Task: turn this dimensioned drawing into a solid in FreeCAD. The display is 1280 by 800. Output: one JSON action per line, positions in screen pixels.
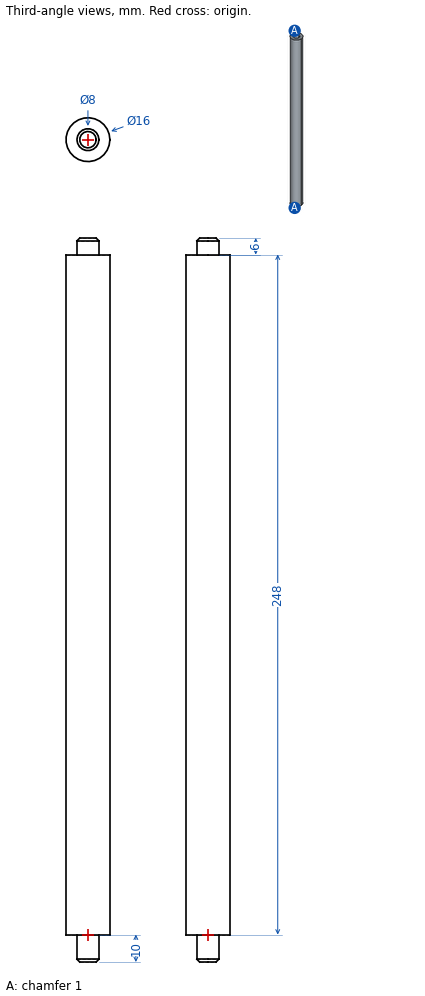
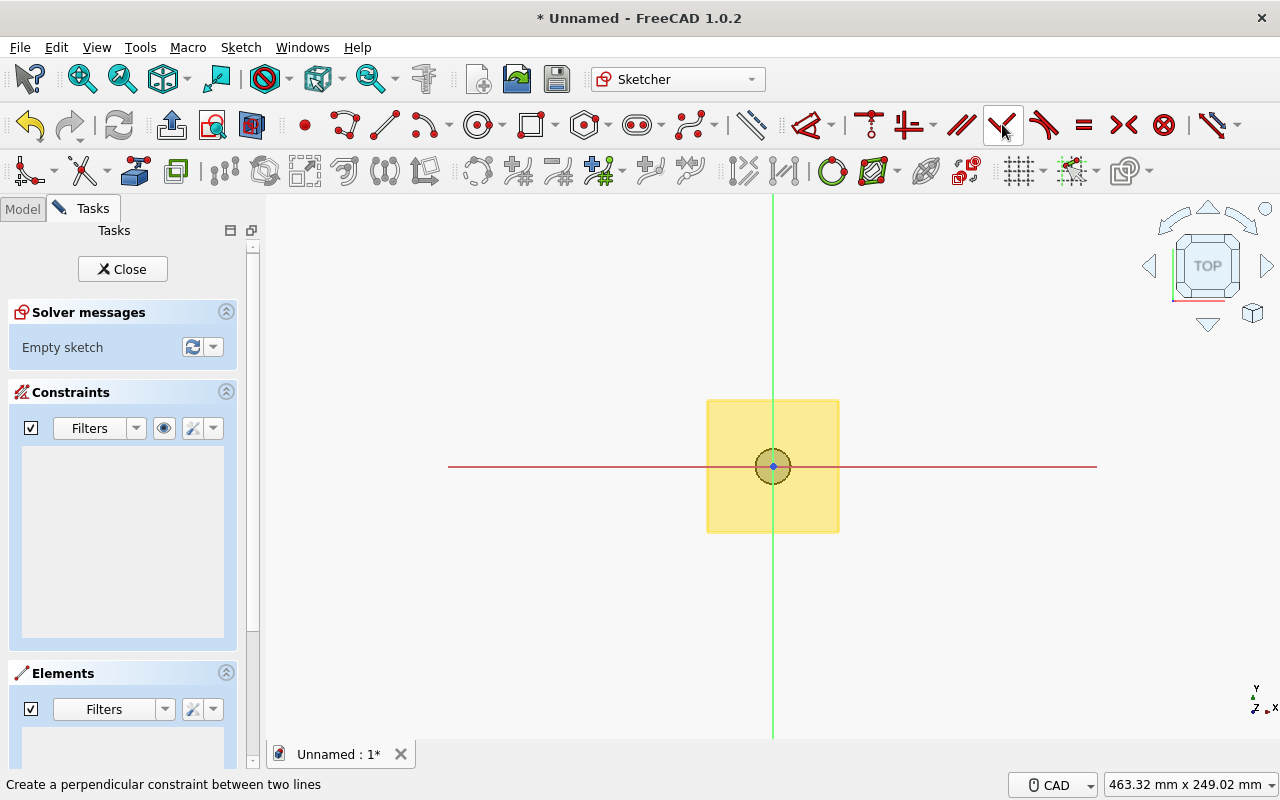
{"action": "scroll", "coordinate": [777, 466], "scroll_direction": "up", "scroll_amount": 15}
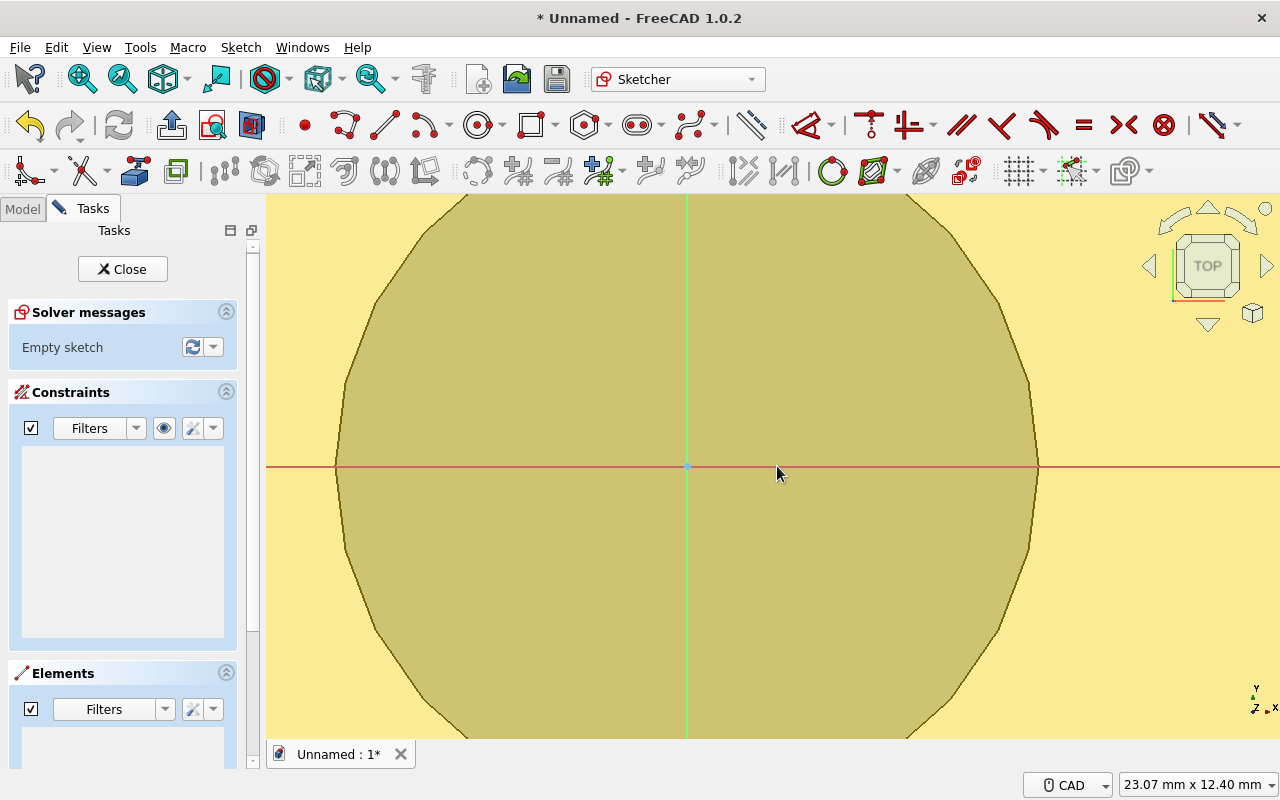
{"action": "key", "text": "g c"}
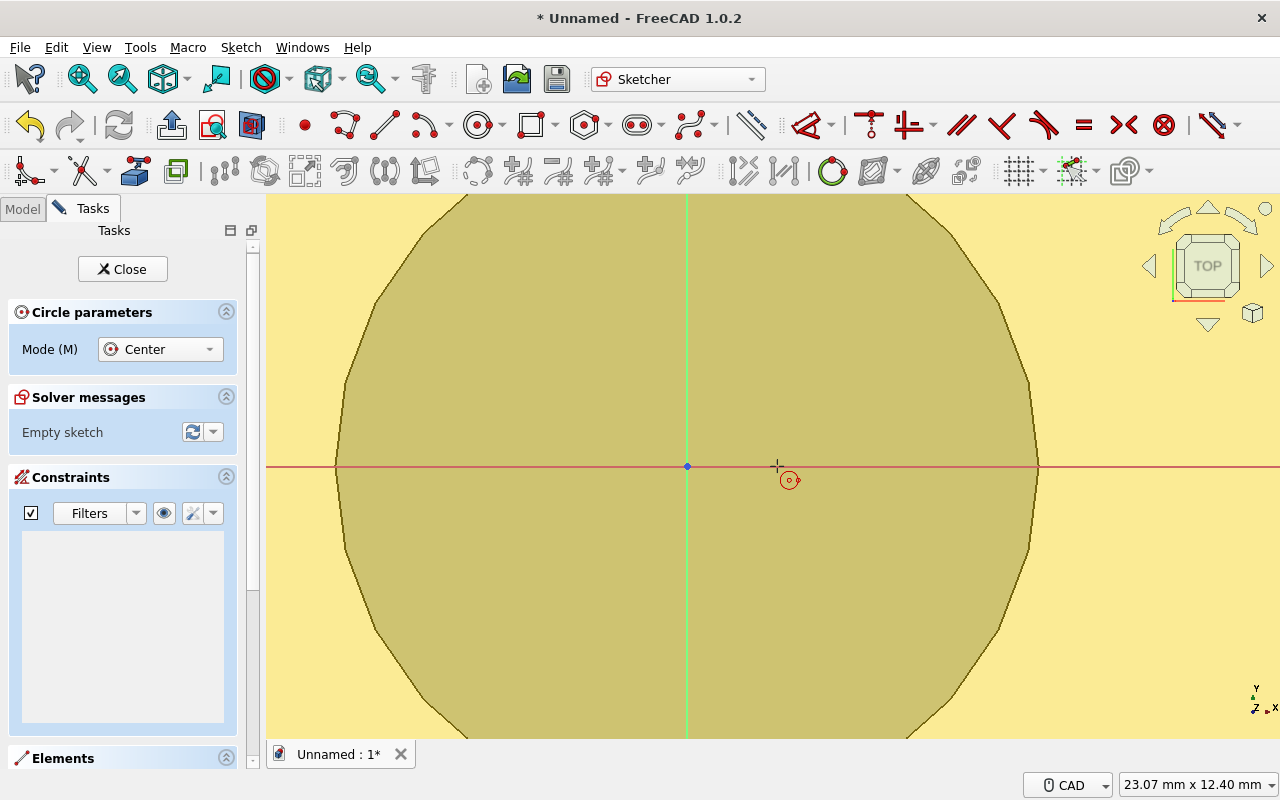
{"action": "left_click", "coordinate": [687, 466]}
{"action": "left_click", "coordinate": [811, 342]}
{"action": "key", "text": "Escape"}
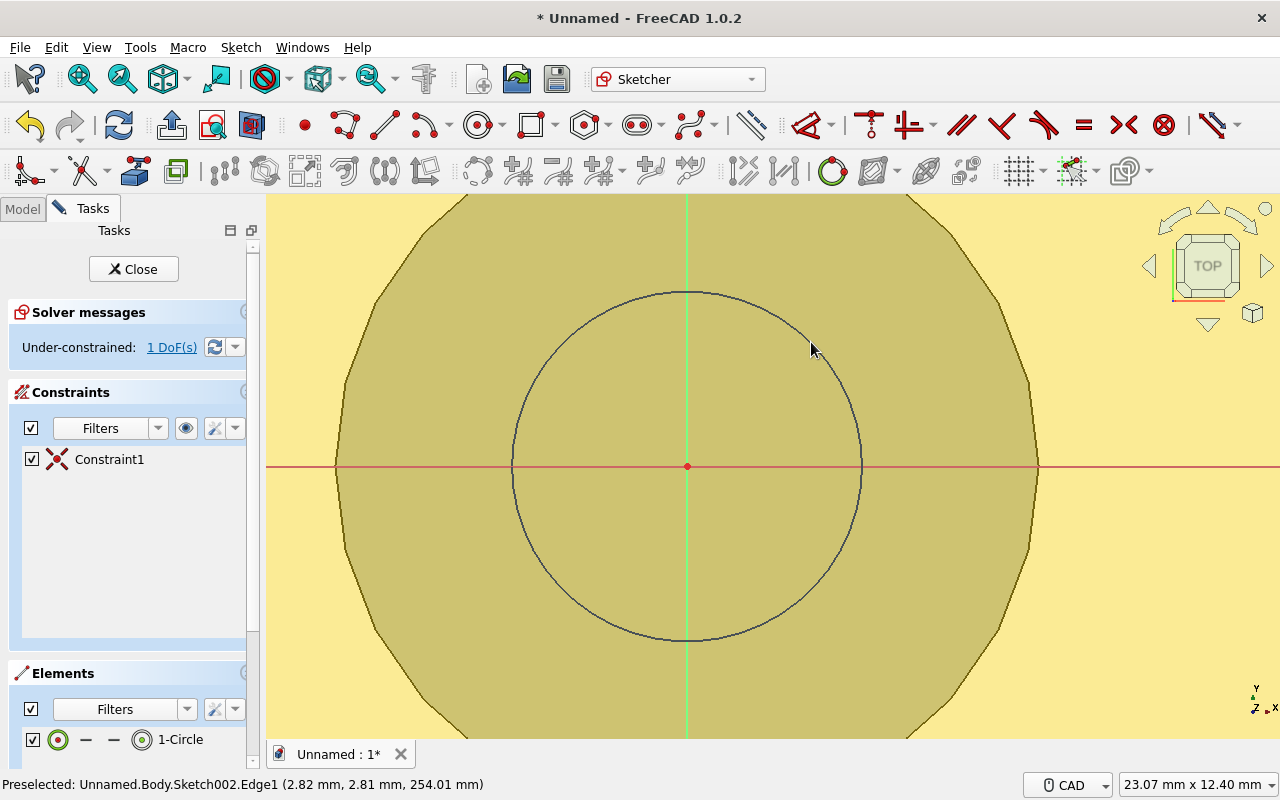
{"action": "left_click", "coordinate": [806, 126]}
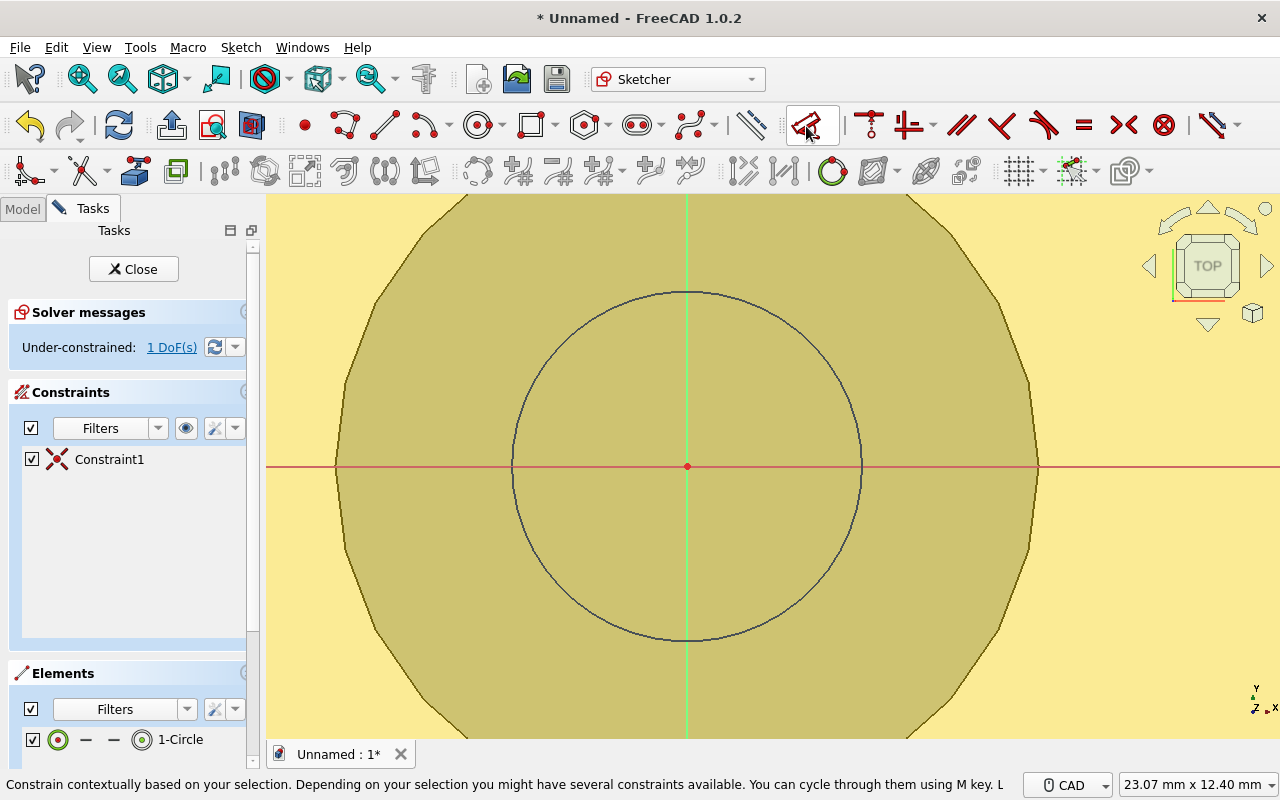
{"action": "left_click", "coordinate": [810, 342]}
{"action": "left_click", "coordinate": [832, 319]}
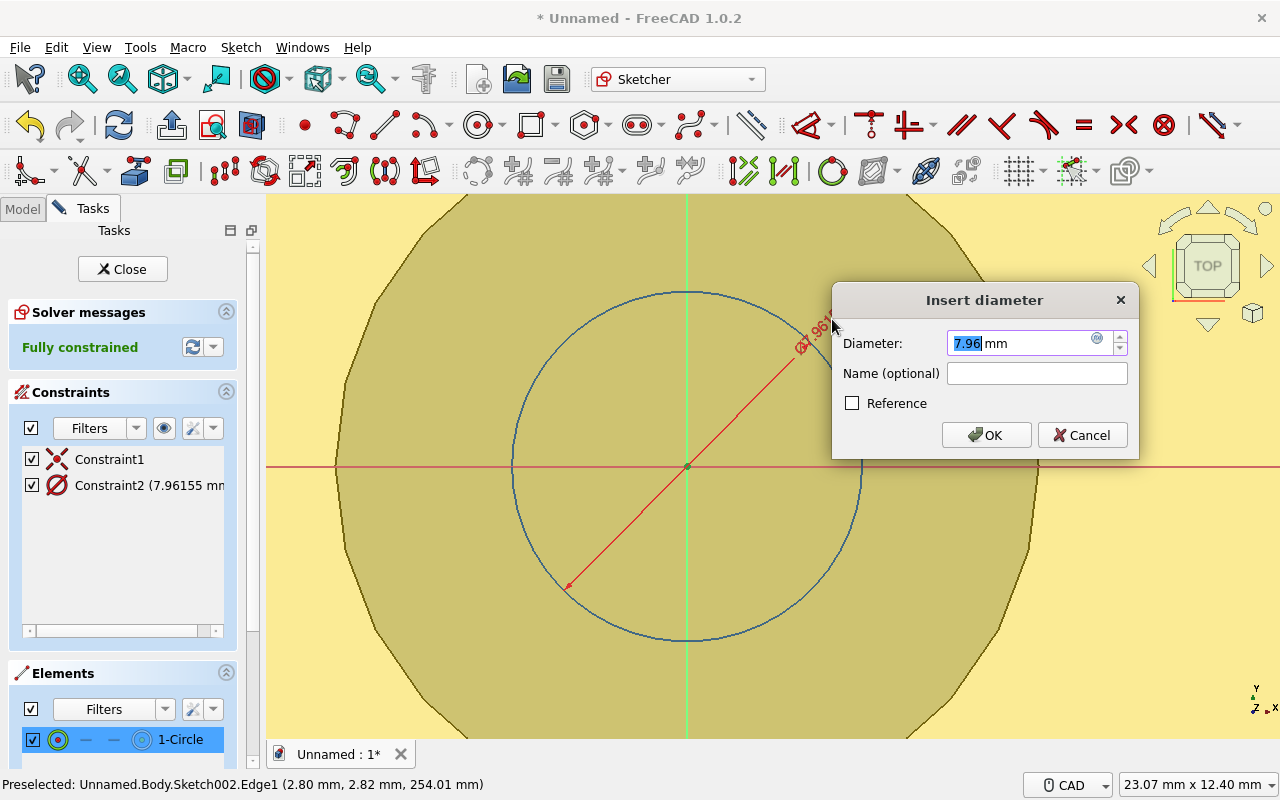
{"action": "type", "text": "8"}
{"action": "key", "text": "Return"}
{"action": "key", "text": "Escape"}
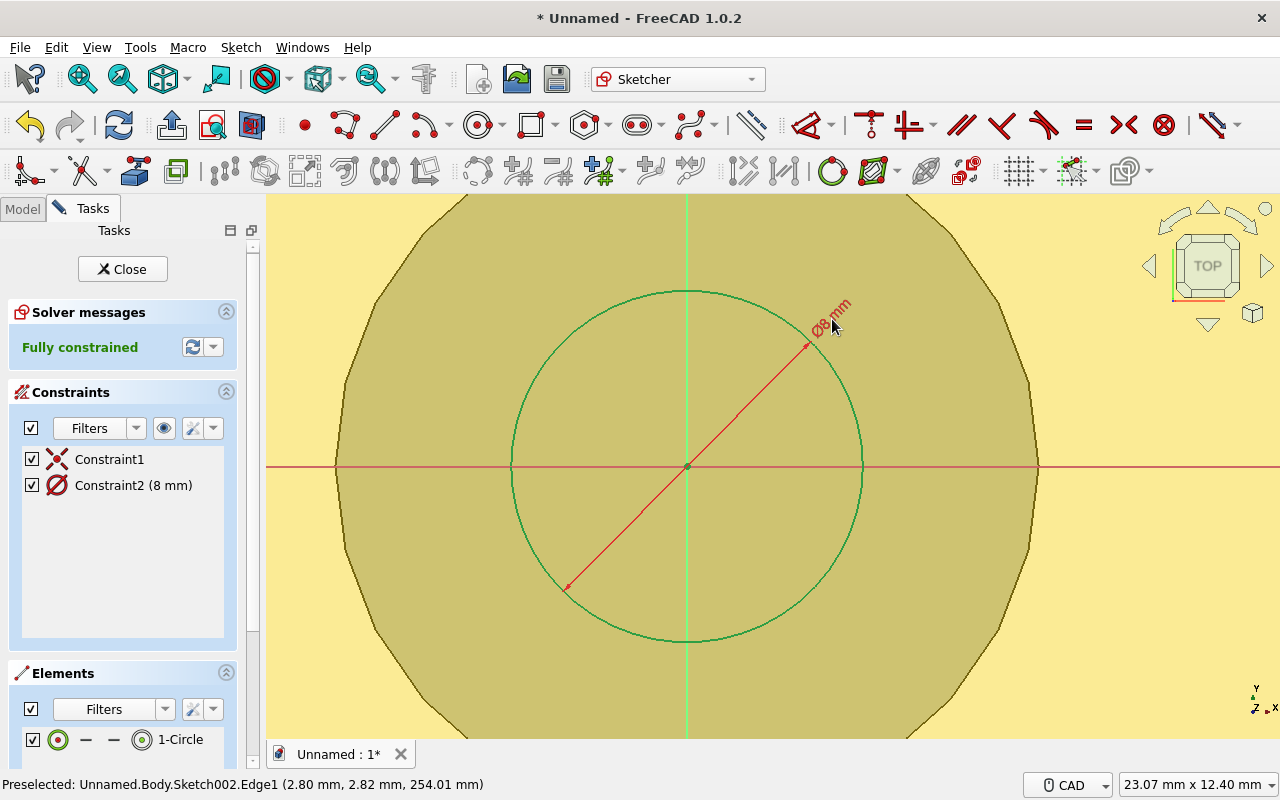
{"action": "left_click", "coordinate": [123, 269]}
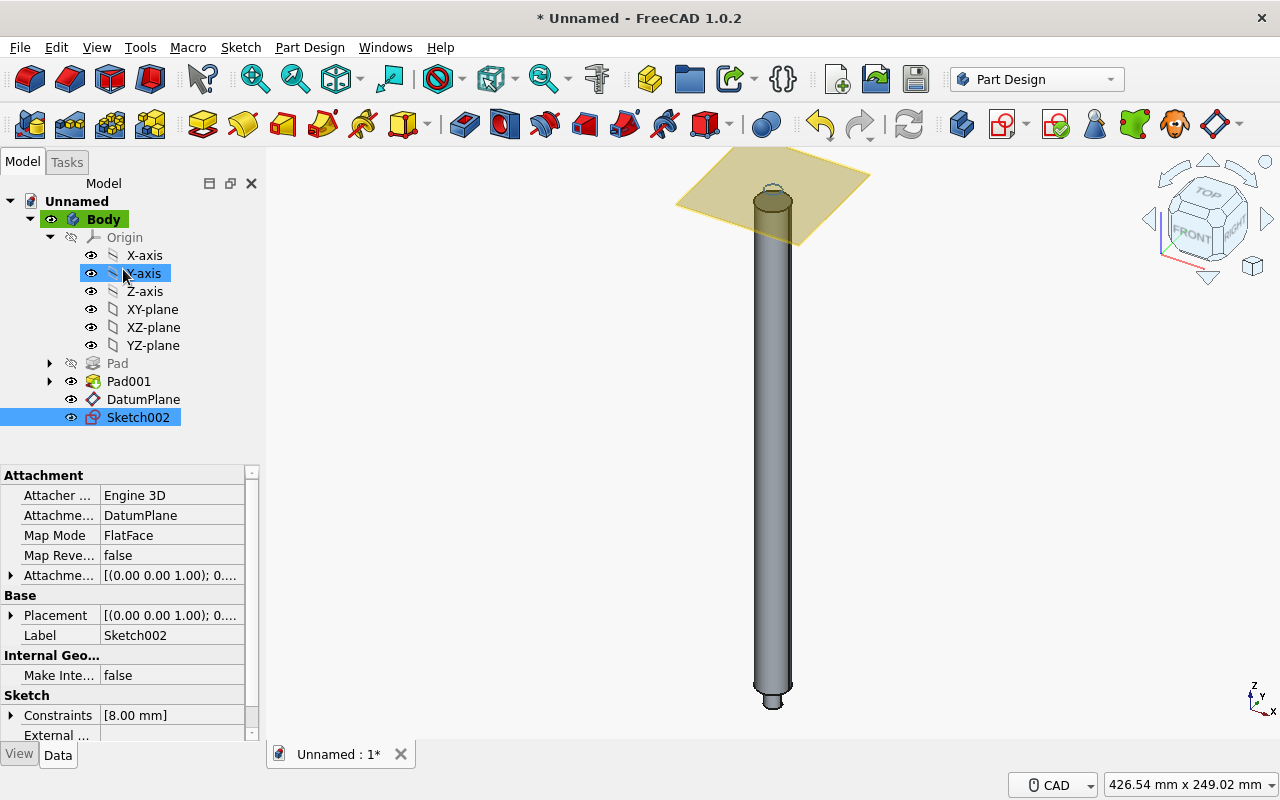
{"action": "left_click", "coordinate": [204, 124]}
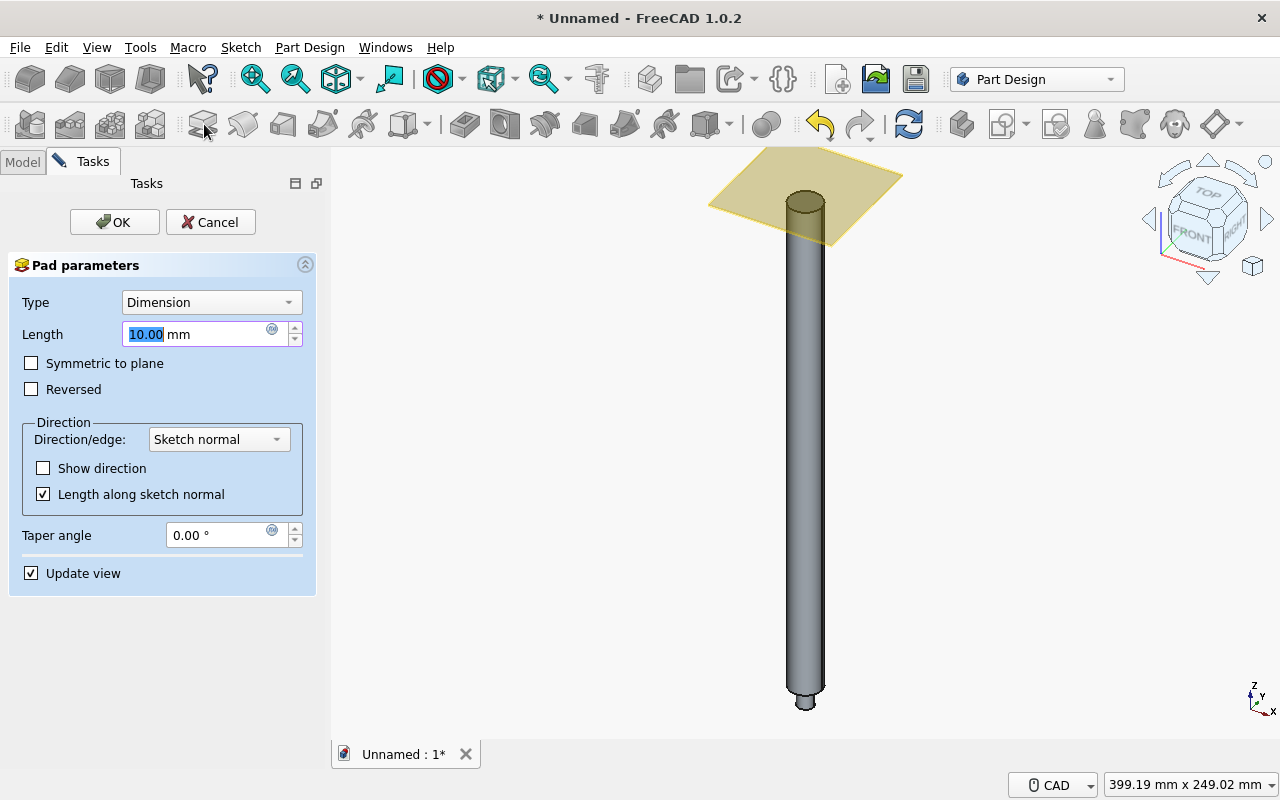
{"action": "type", "text": "6"}
{"action": "key", "text": "Tab"}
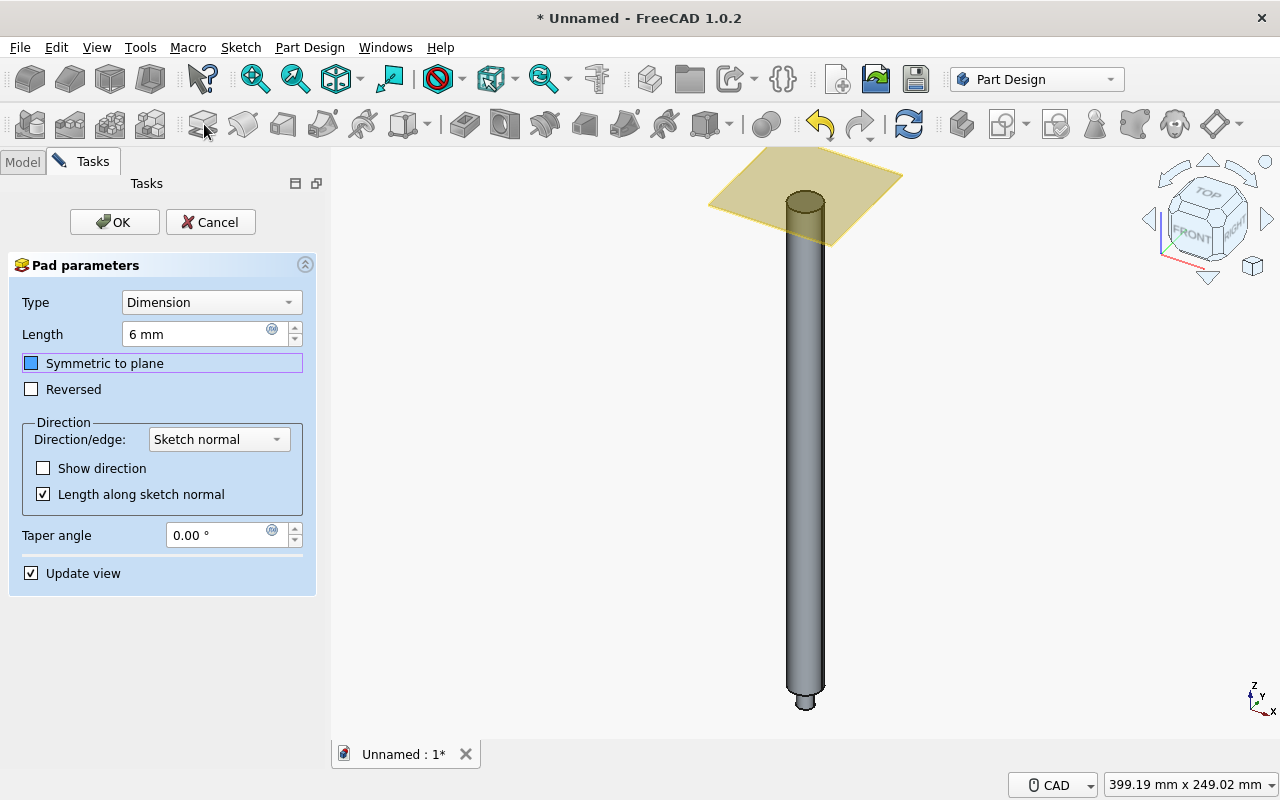
{"action": "left_click", "coordinate": [30, 389]}